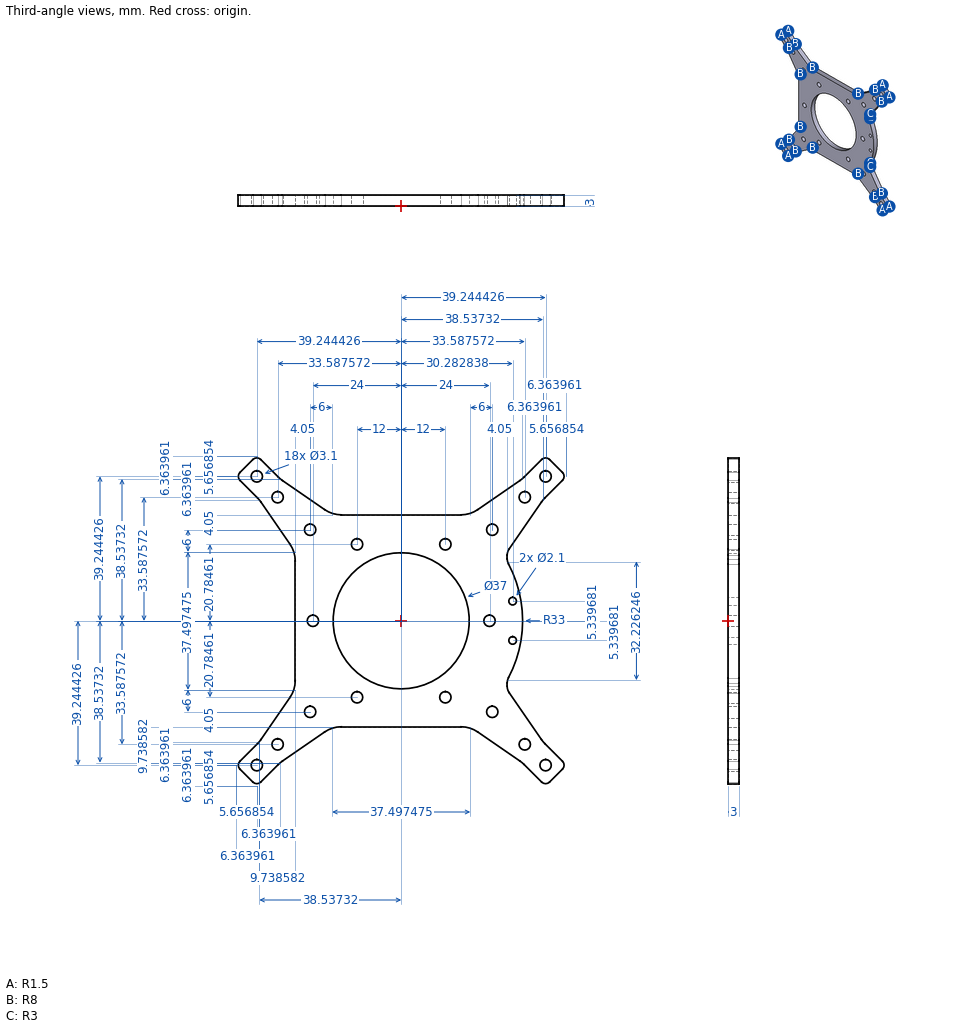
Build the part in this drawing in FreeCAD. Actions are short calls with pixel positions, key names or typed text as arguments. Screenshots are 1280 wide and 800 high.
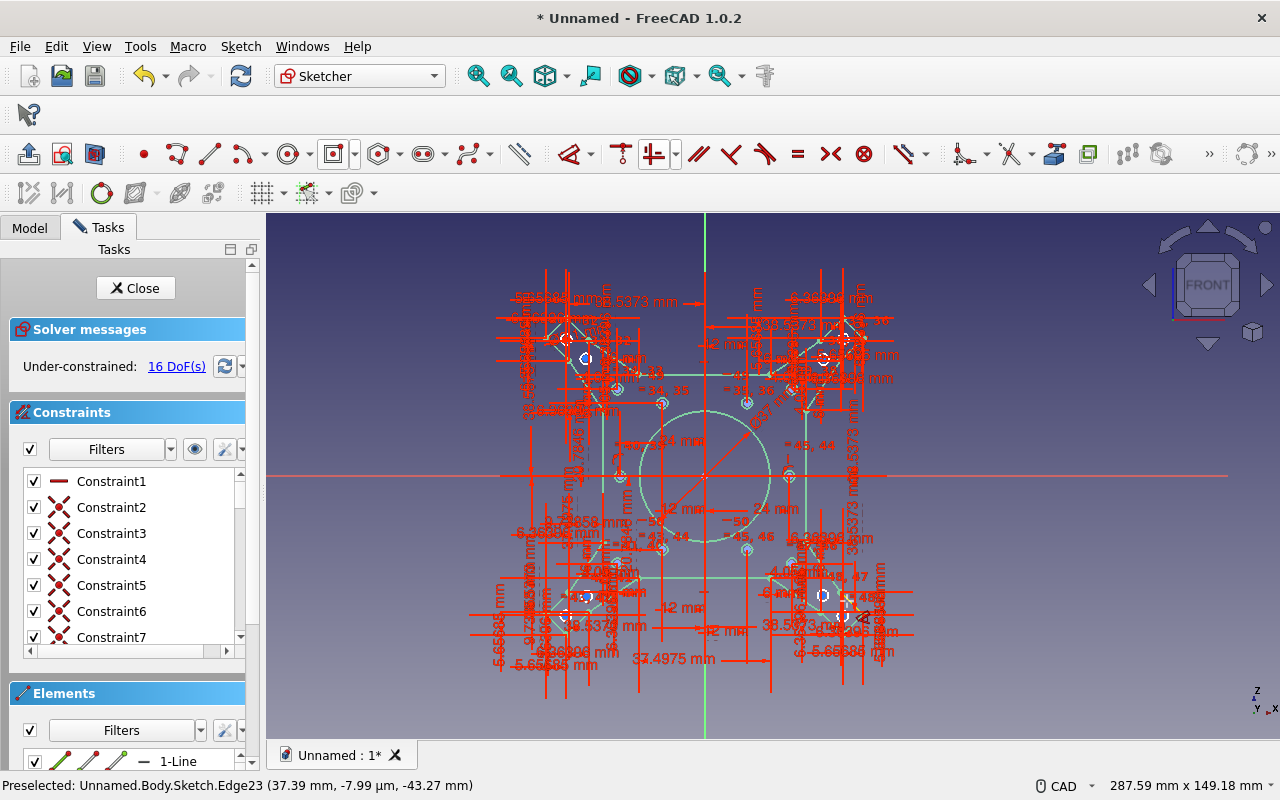
click(566, 339)
click(635, 281)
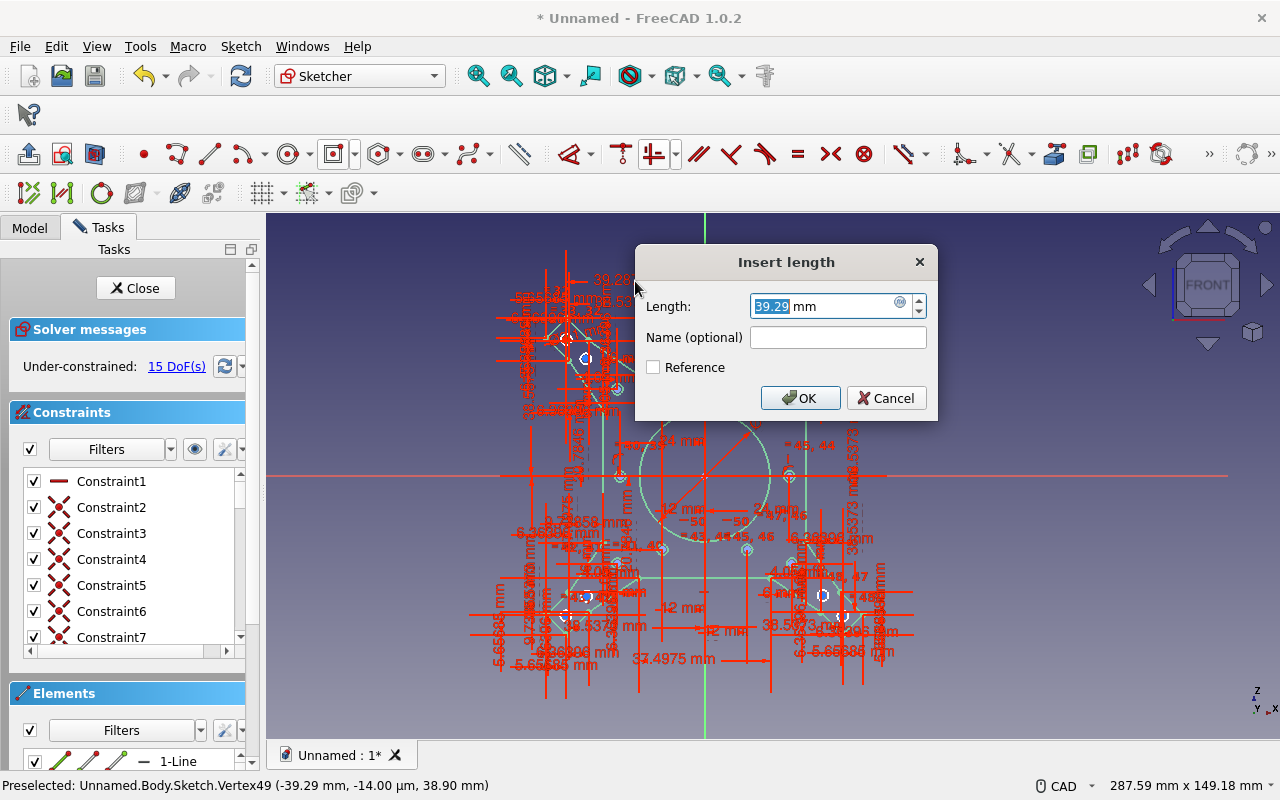
text(39.244426)
key(Return)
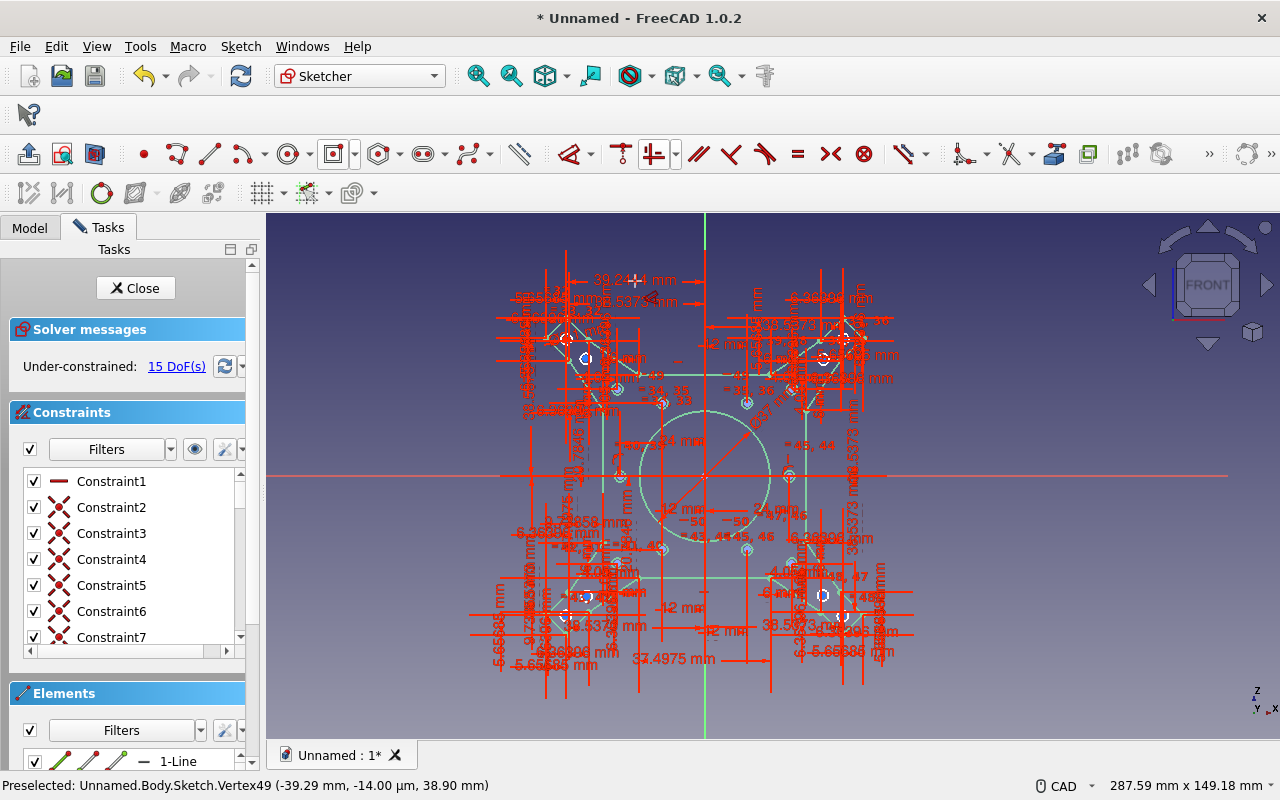
click(566, 339)
click(508, 439)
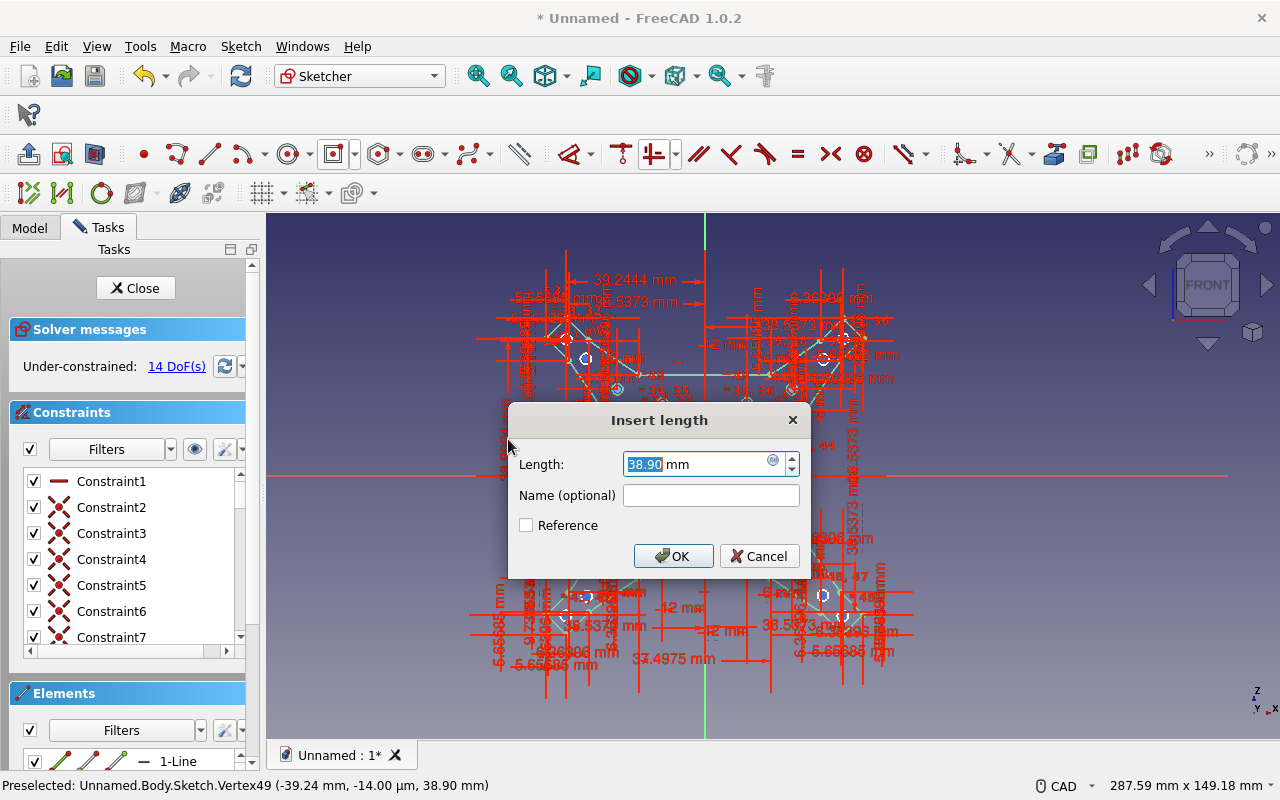
text(39.244426)
key(Return)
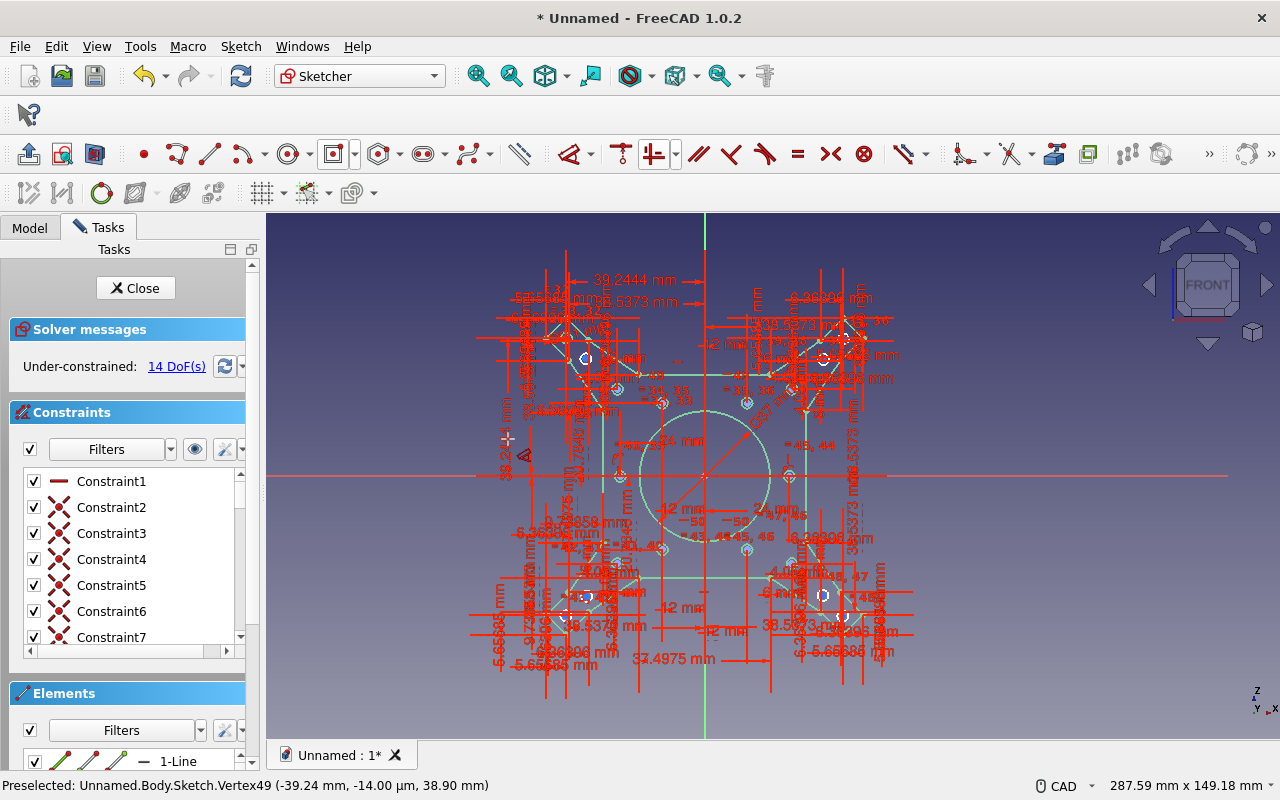
click(586, 359)
click(687, 325)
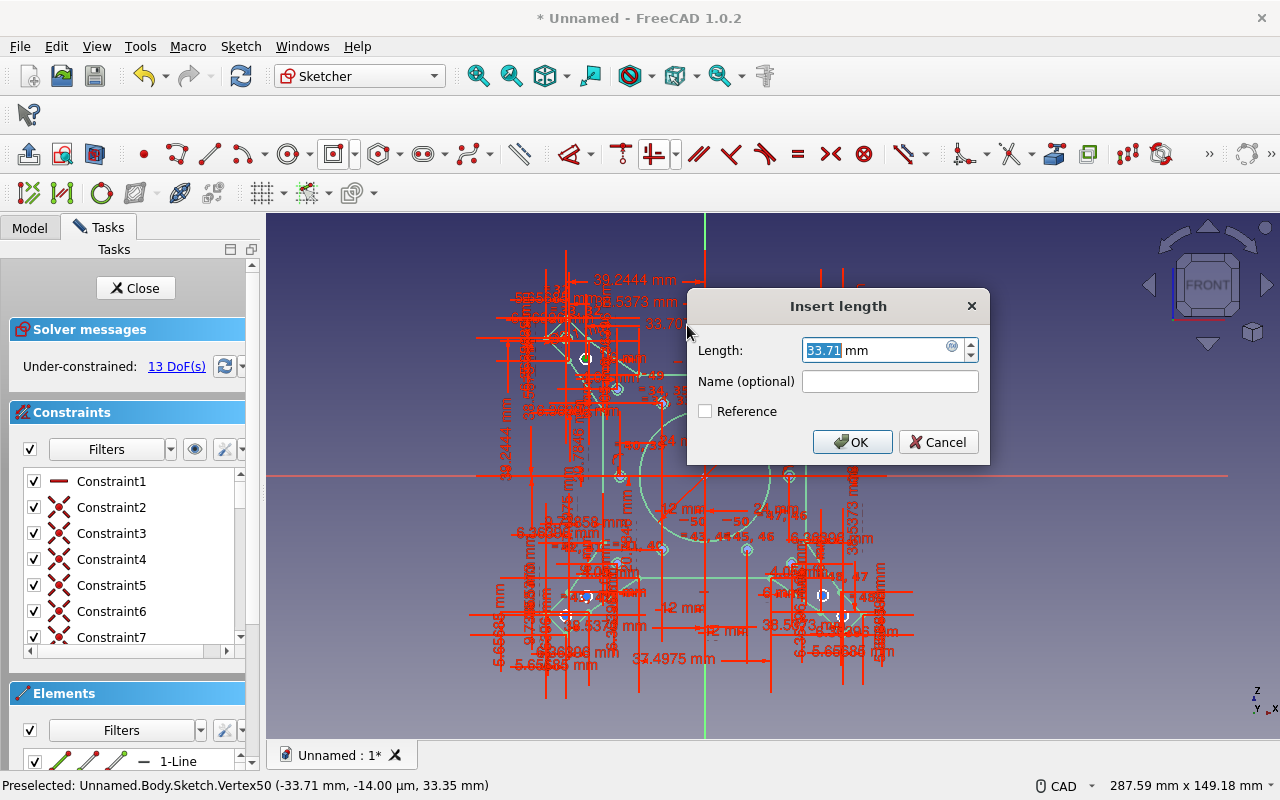
text(33.587572)
key(Return)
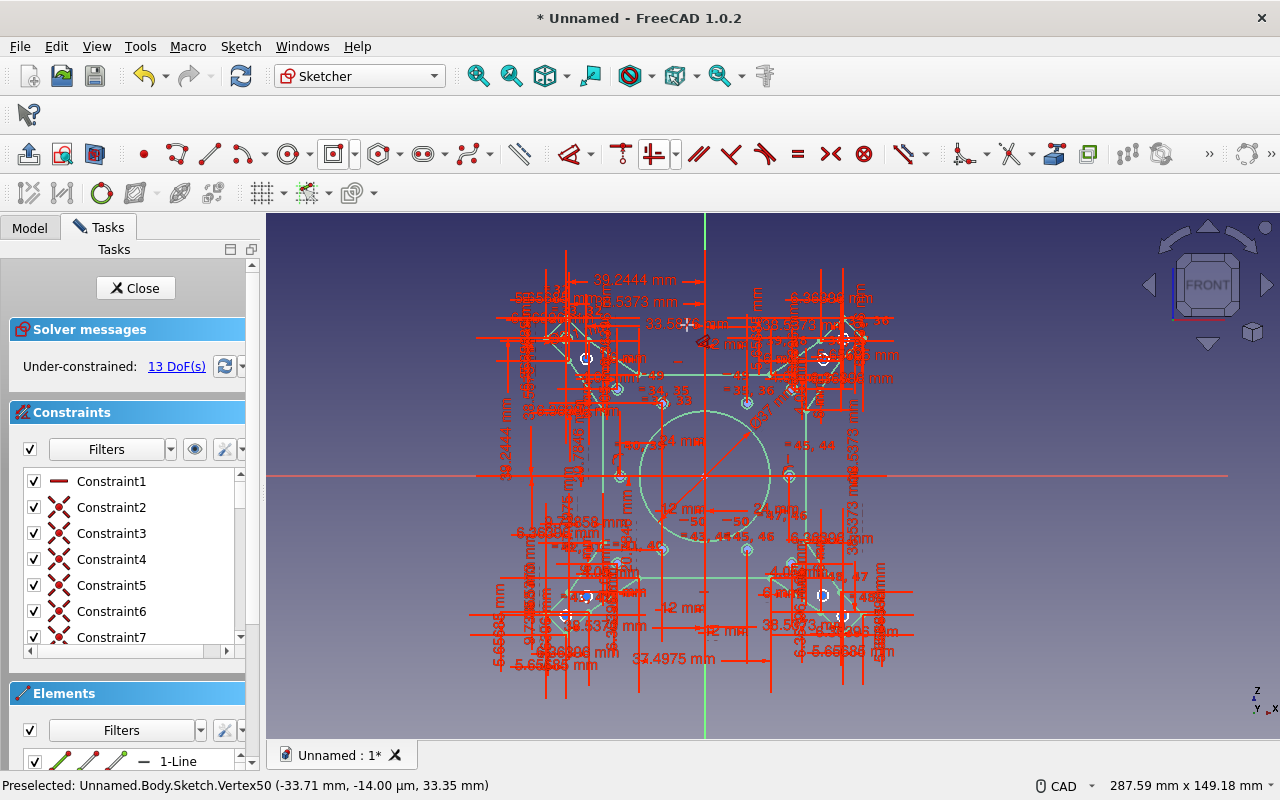
click(586, 359)
click(504, 418)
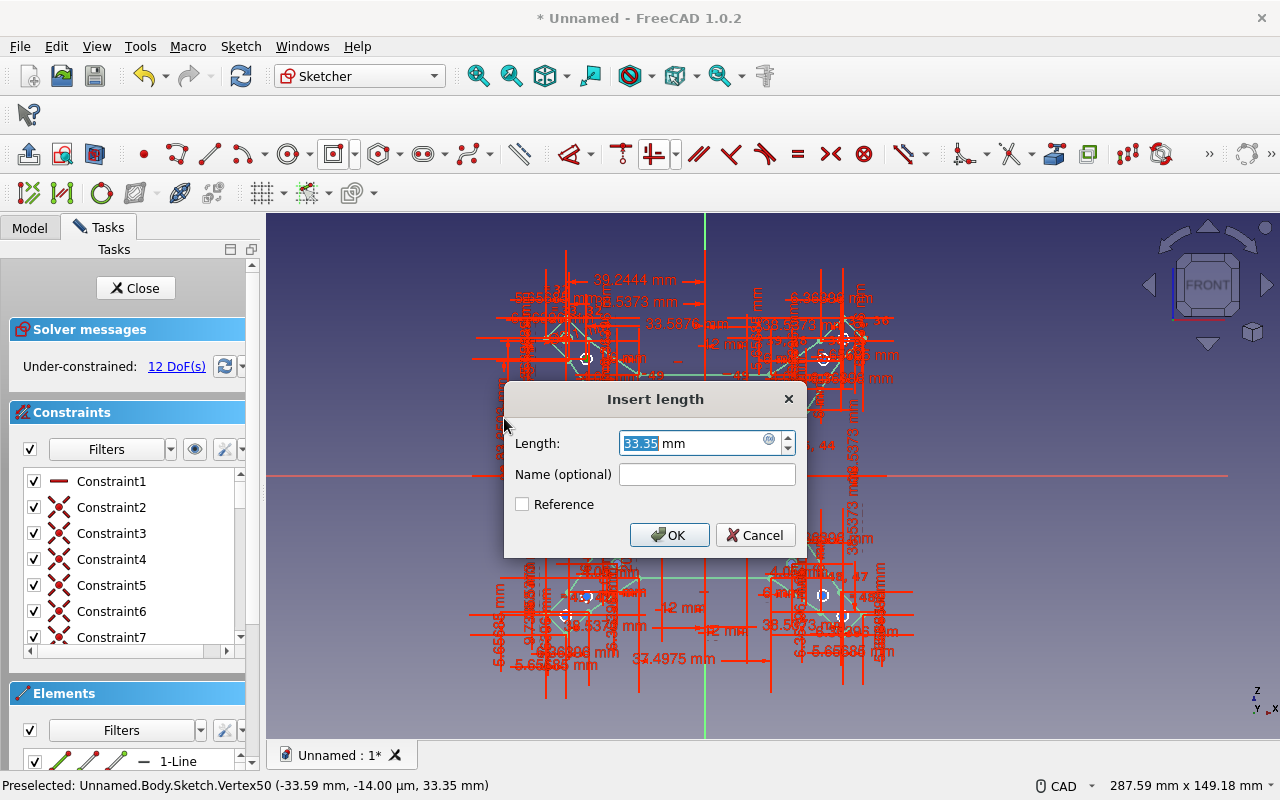
text(33.587572)
key(Return)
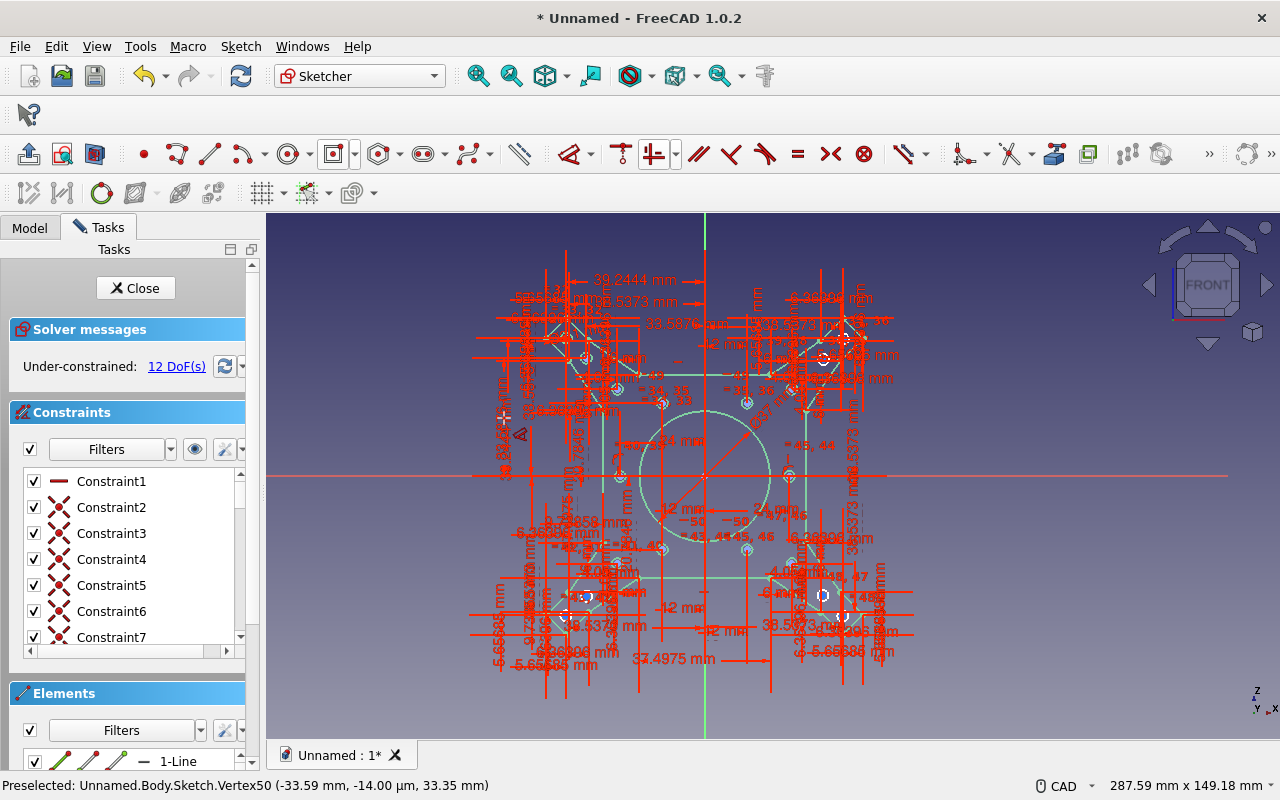
click(843, 339)
click(742, 281)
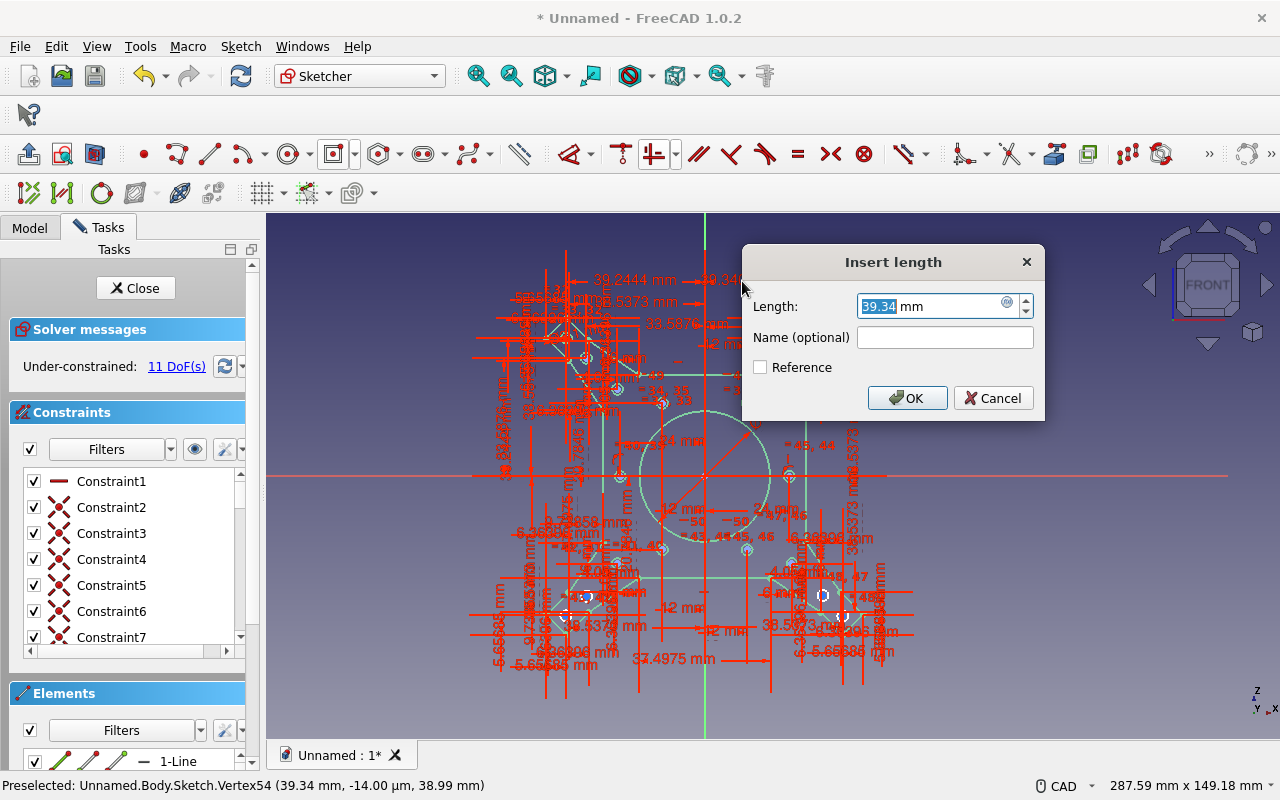
text(39.244426)
key(Return)